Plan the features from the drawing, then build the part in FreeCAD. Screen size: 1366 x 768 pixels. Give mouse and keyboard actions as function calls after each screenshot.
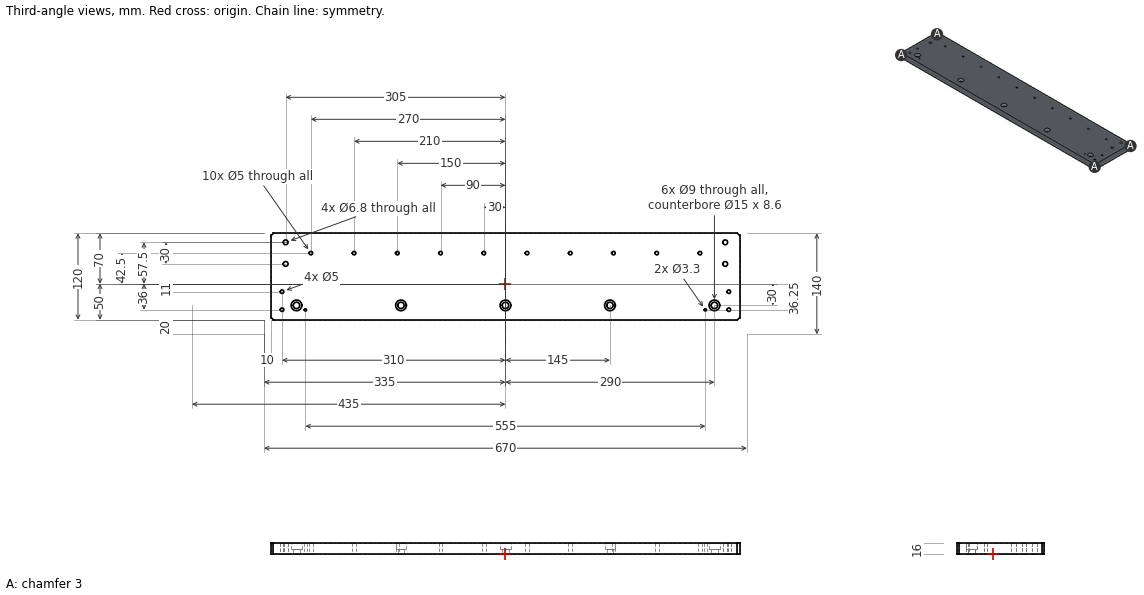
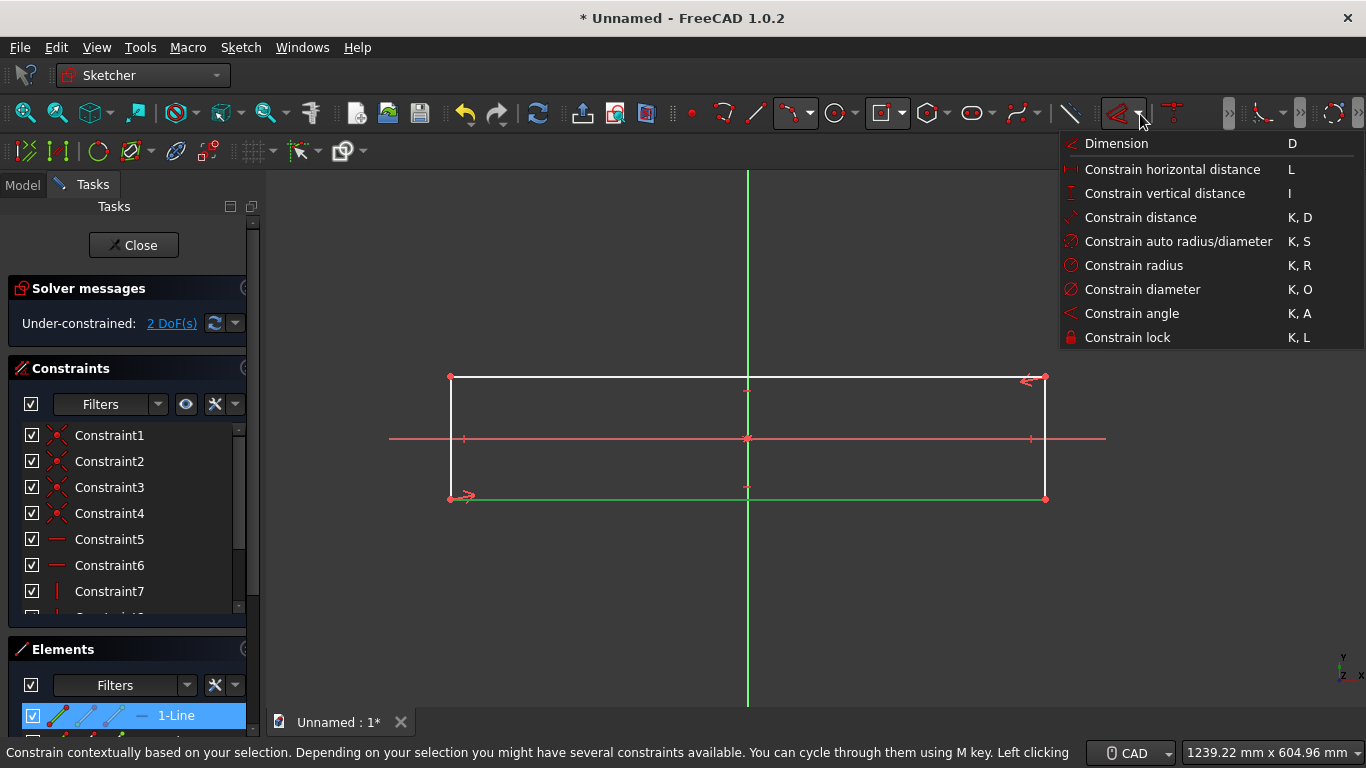
click(1212, 169)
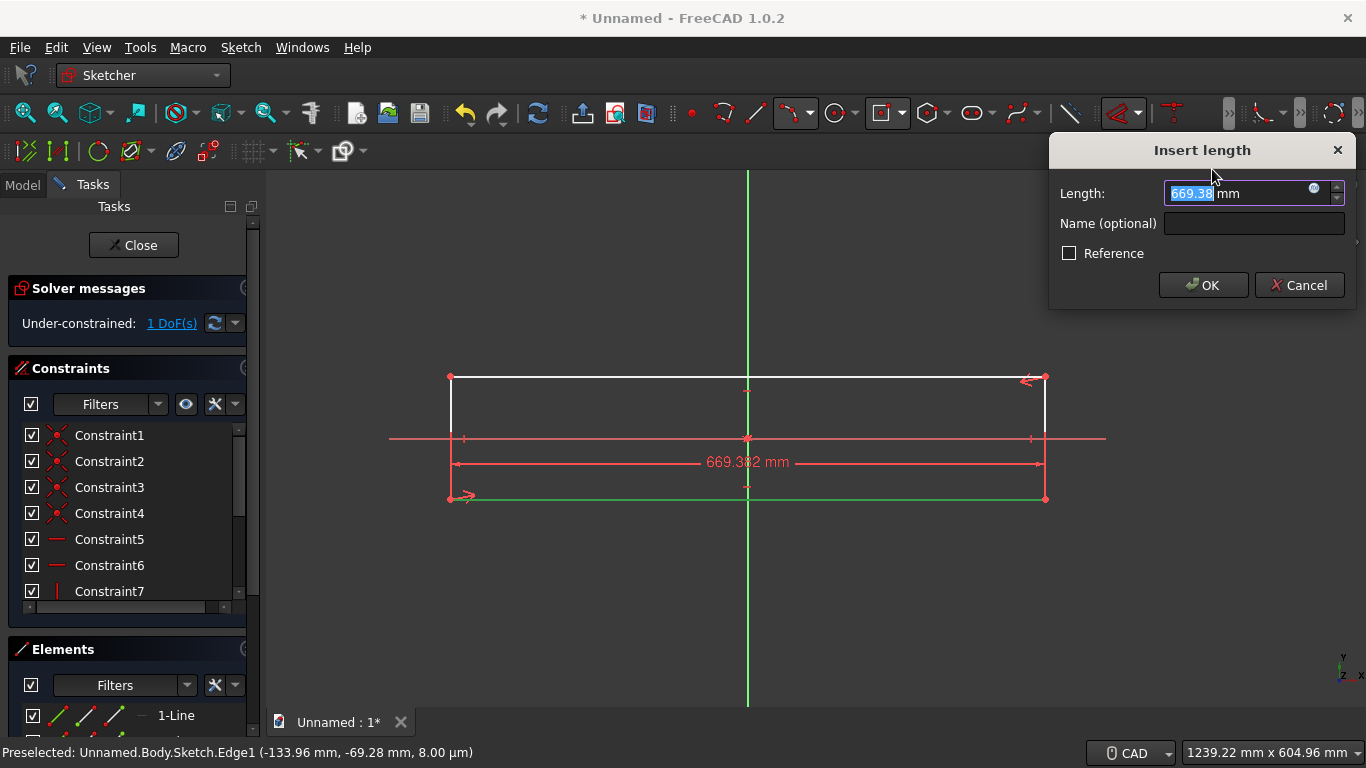
text(670)
key(Return)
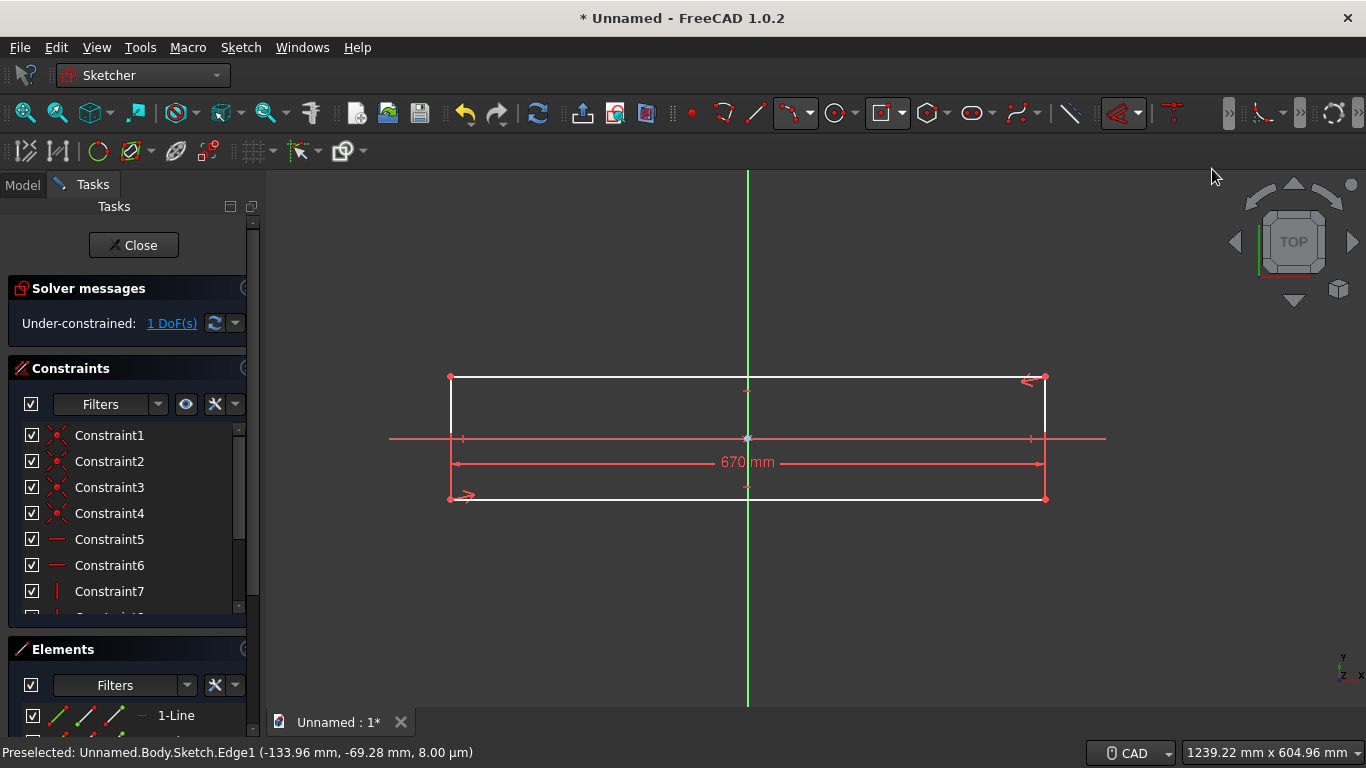
click(1045, 463)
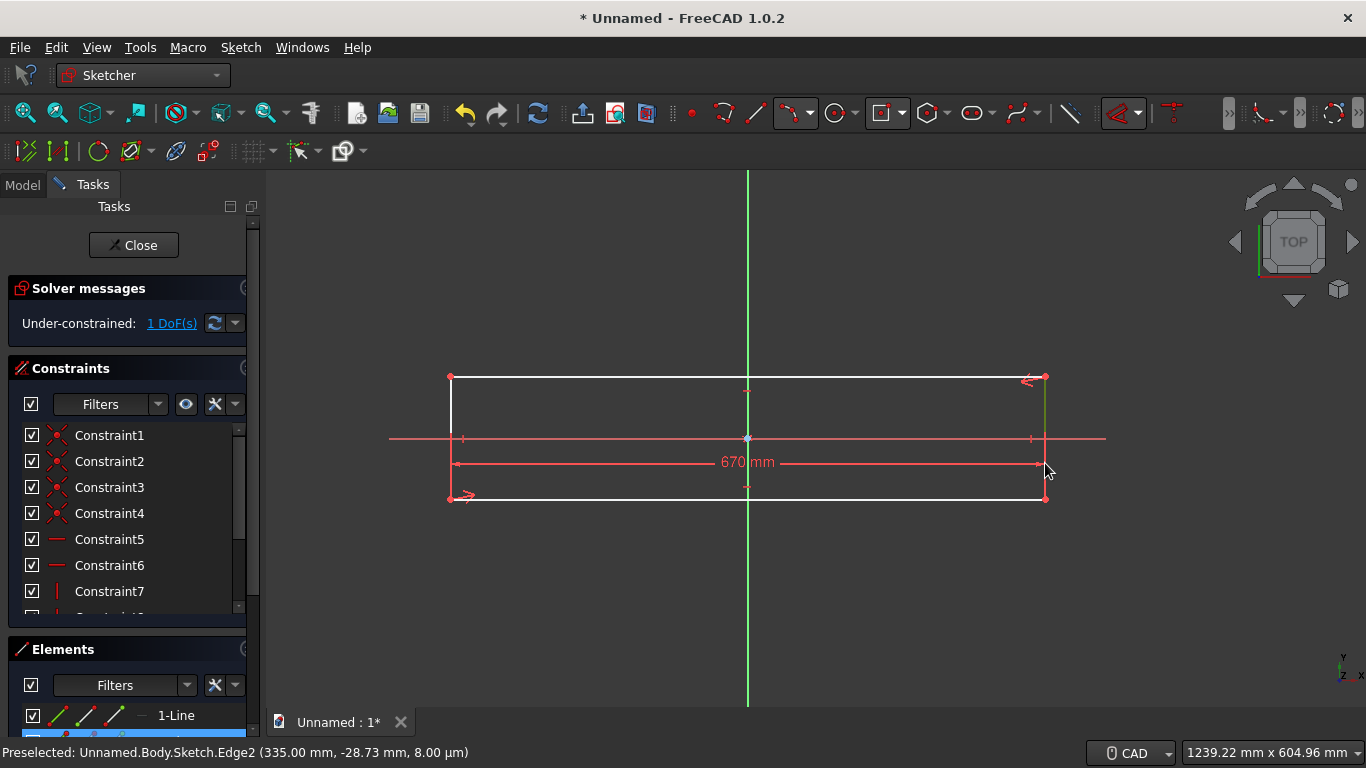
key(i)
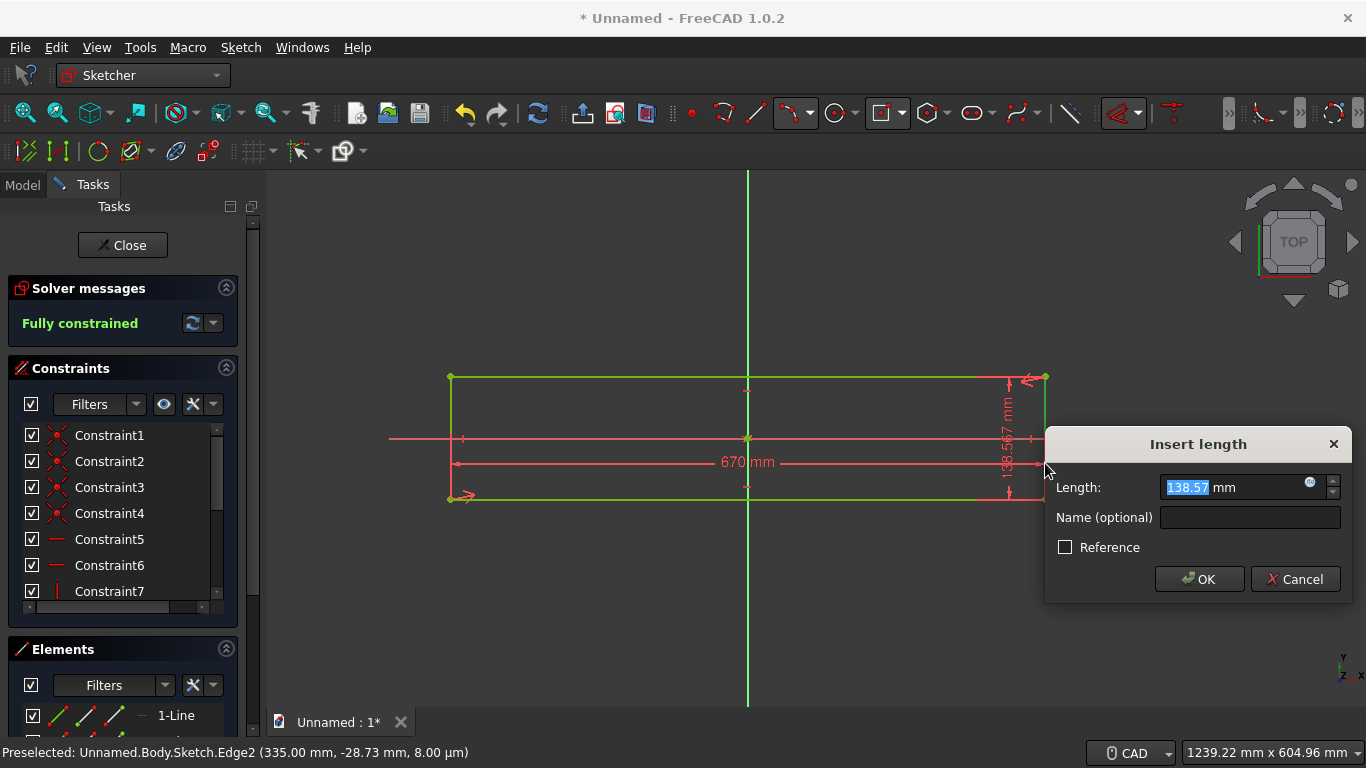
text(140)
key(Return)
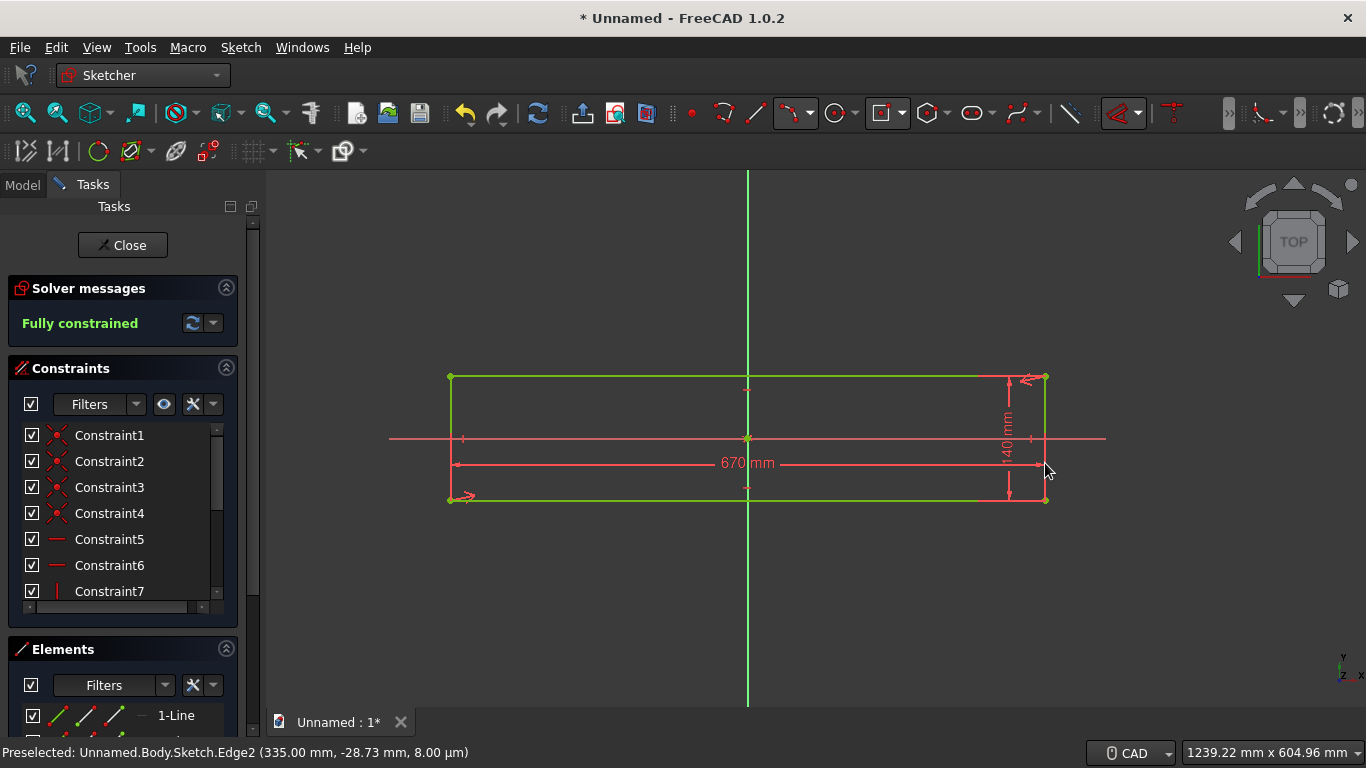
click(123, 245)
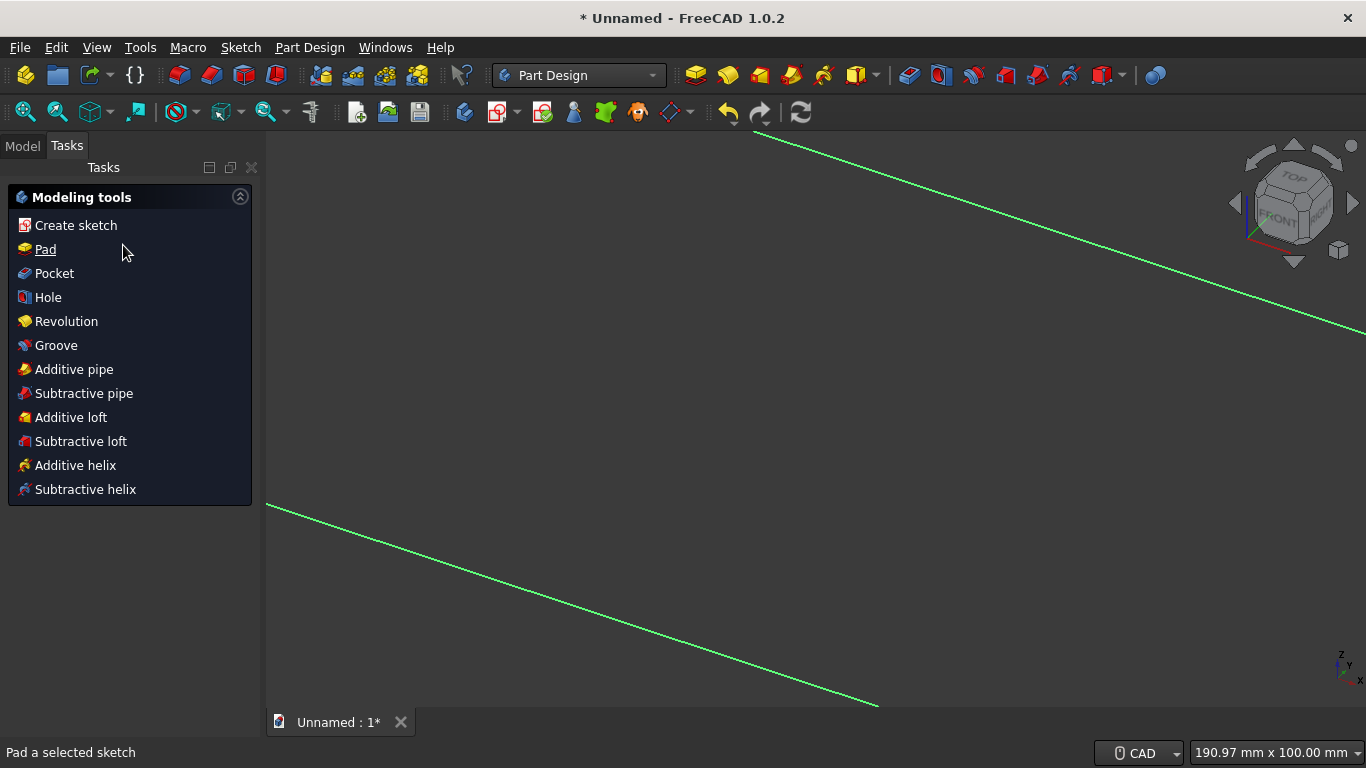
click(696, 76)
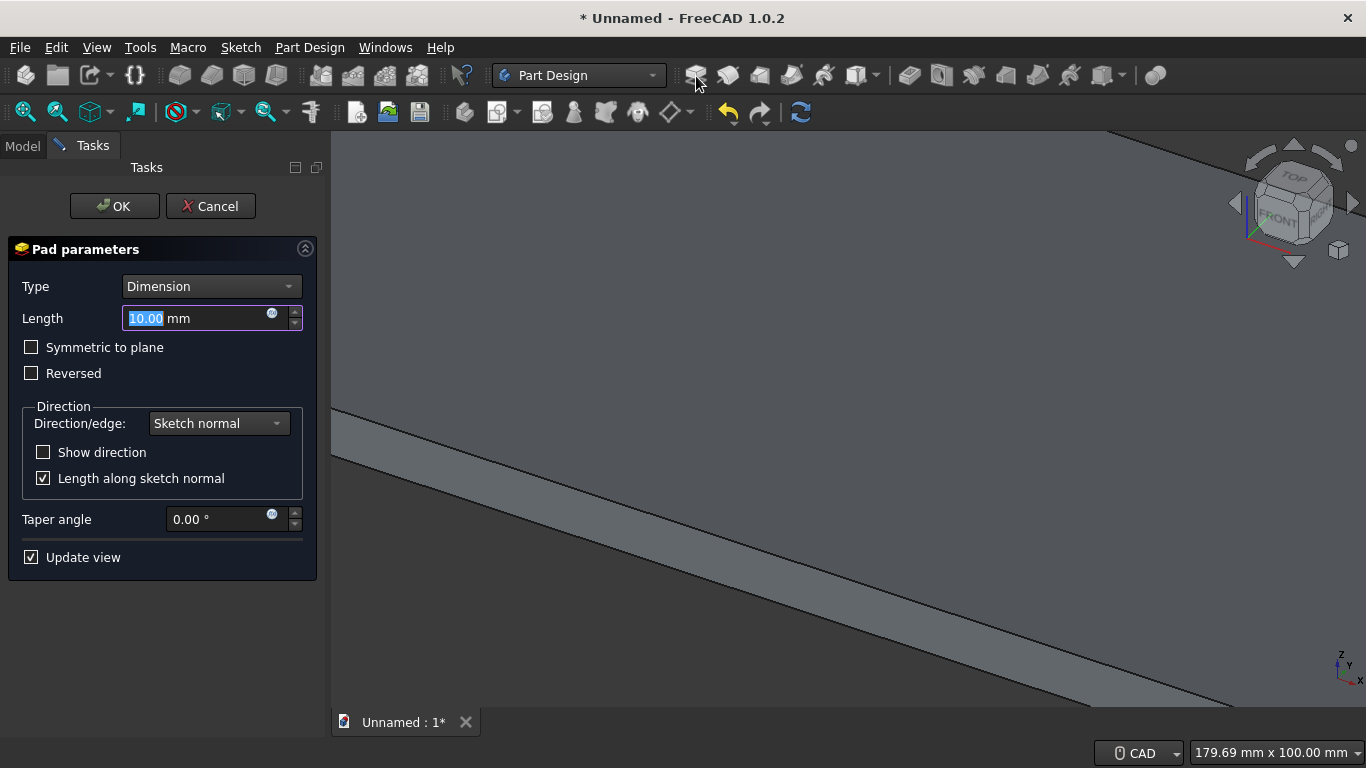
text(16)
key(Tab)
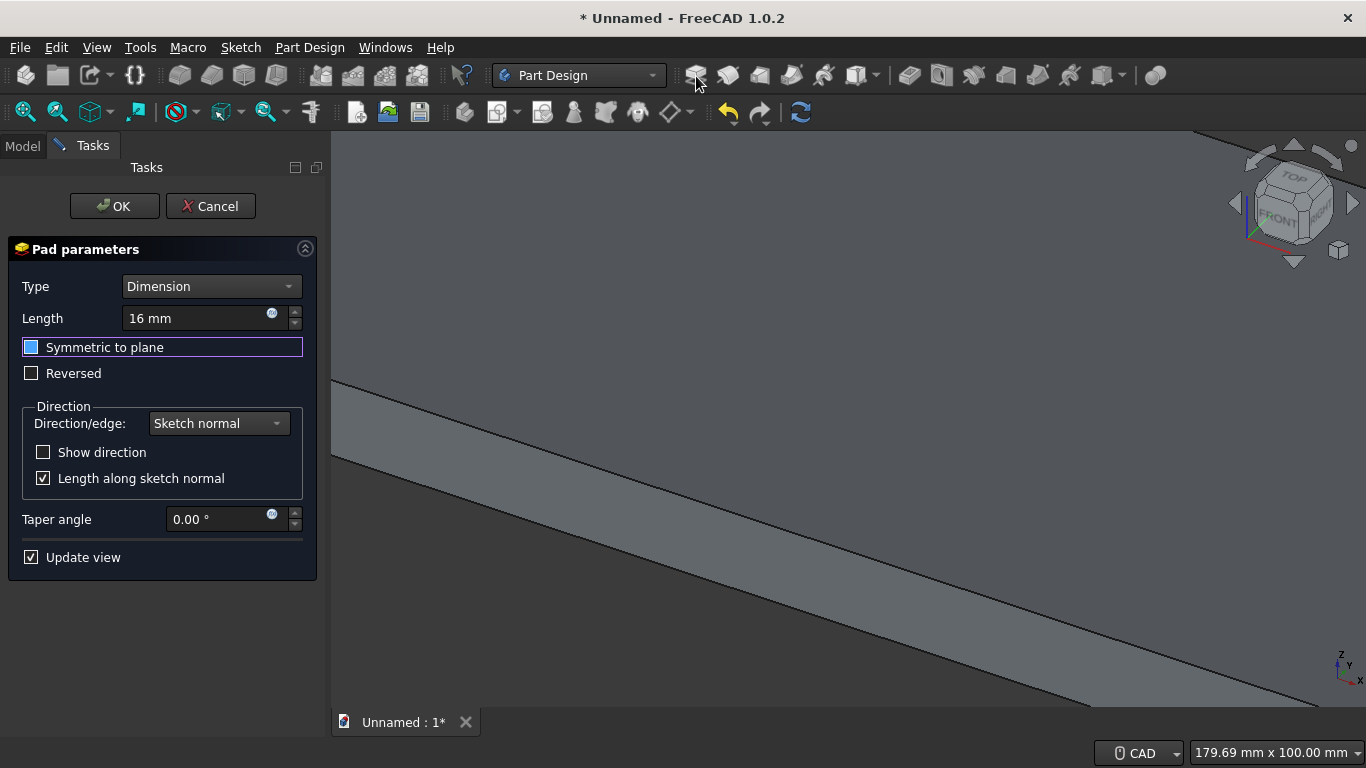
click(115, 206)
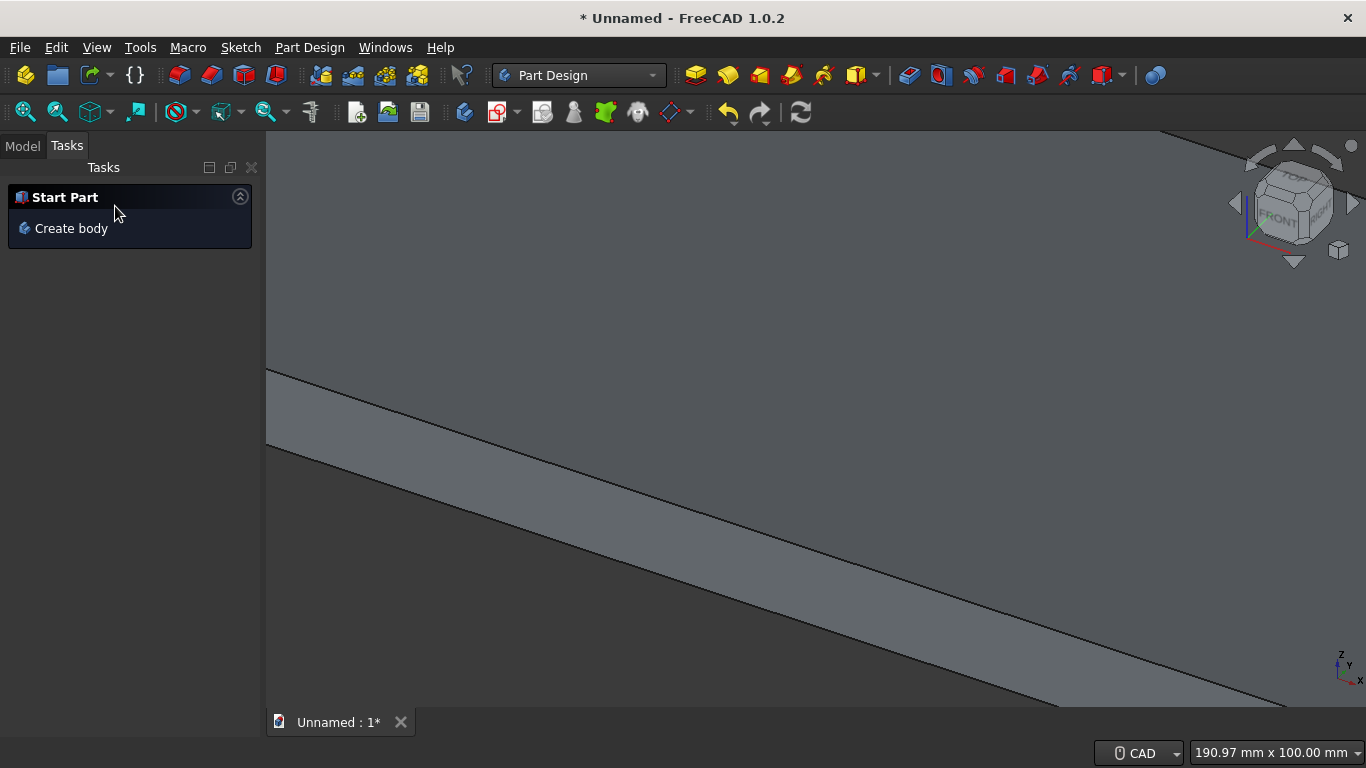
click(26, 112)